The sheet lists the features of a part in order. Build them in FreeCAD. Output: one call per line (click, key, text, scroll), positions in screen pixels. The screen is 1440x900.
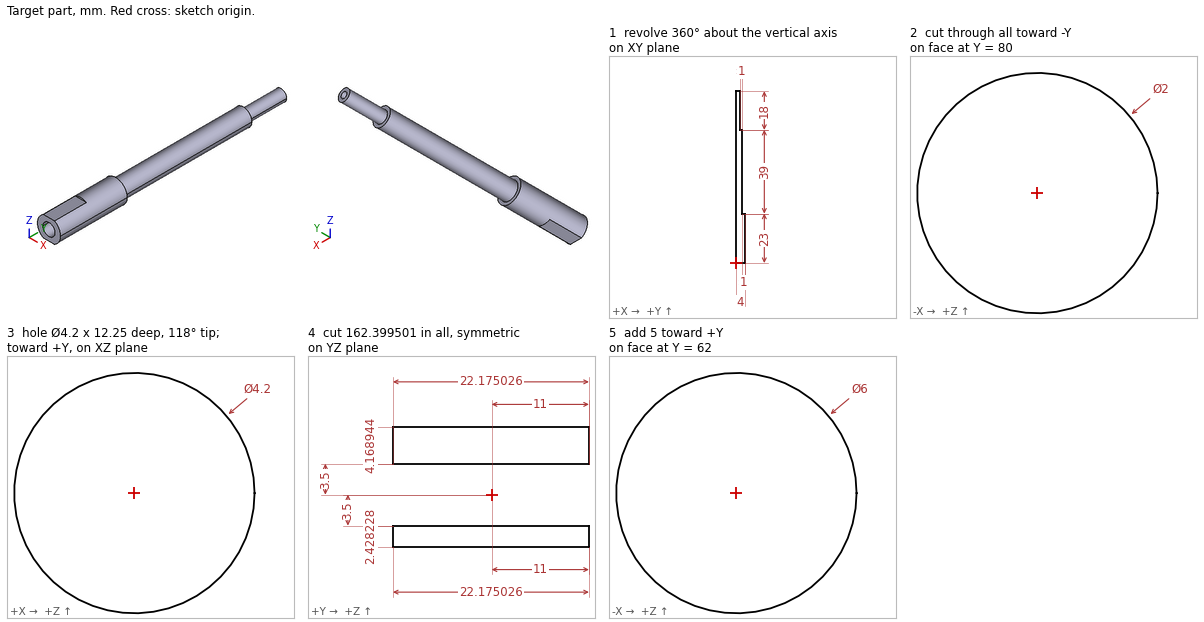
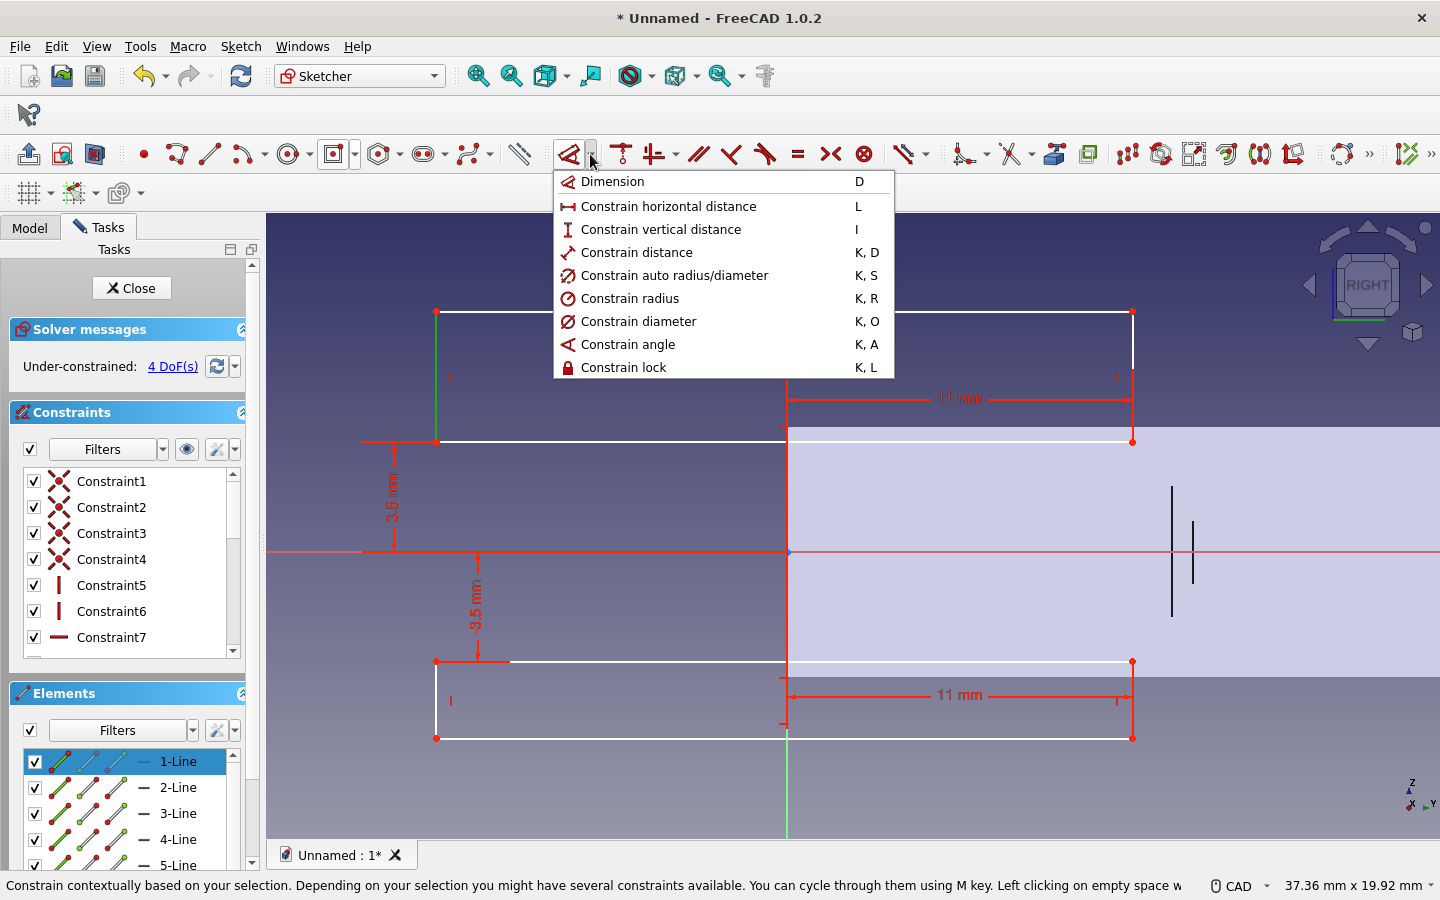
click(724, 230)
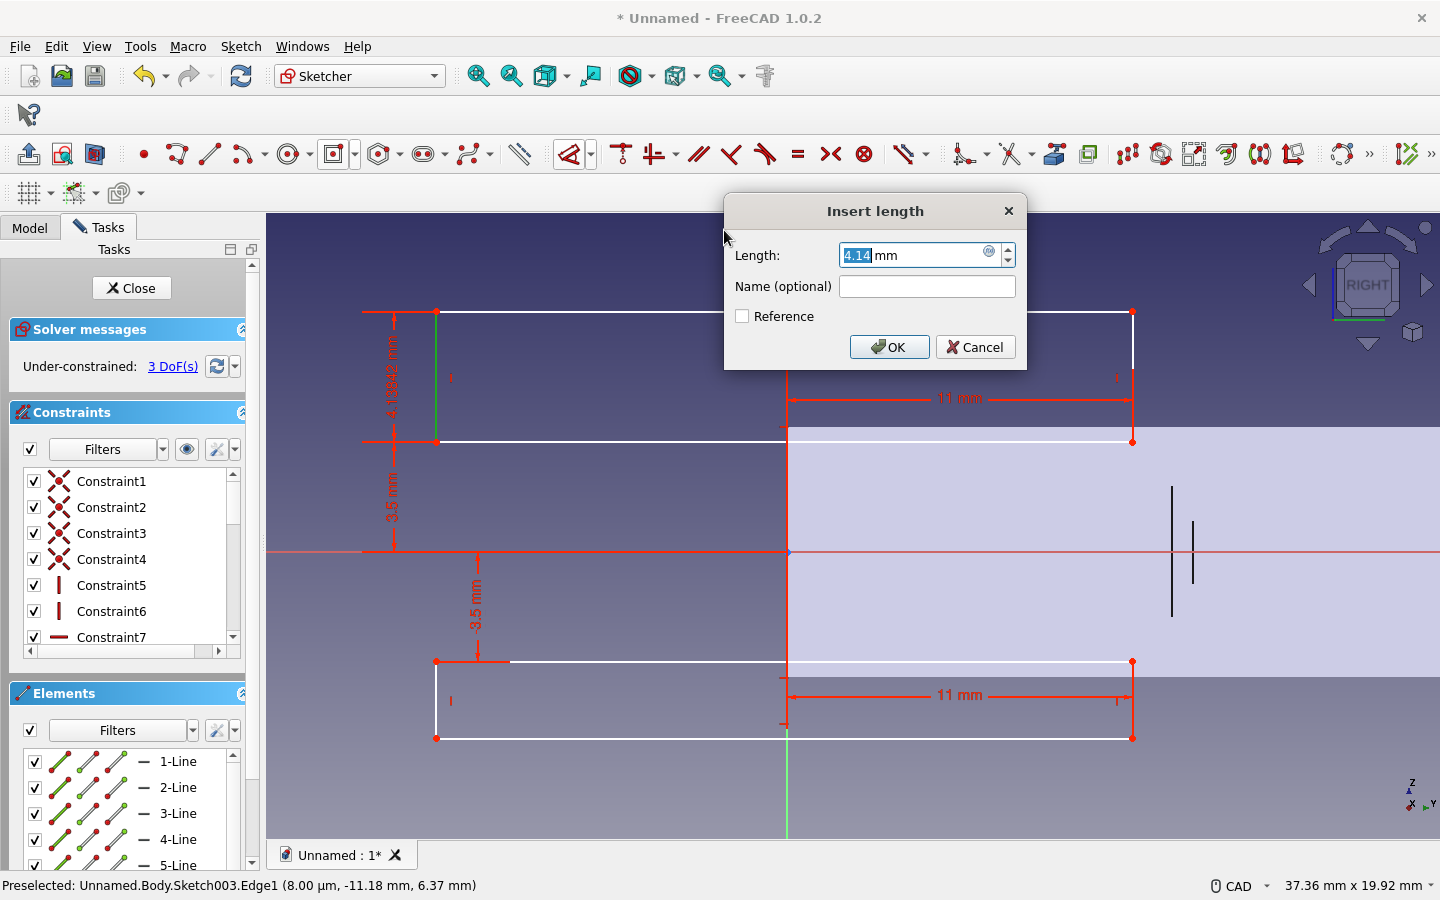
text(4.168944)
key(Return)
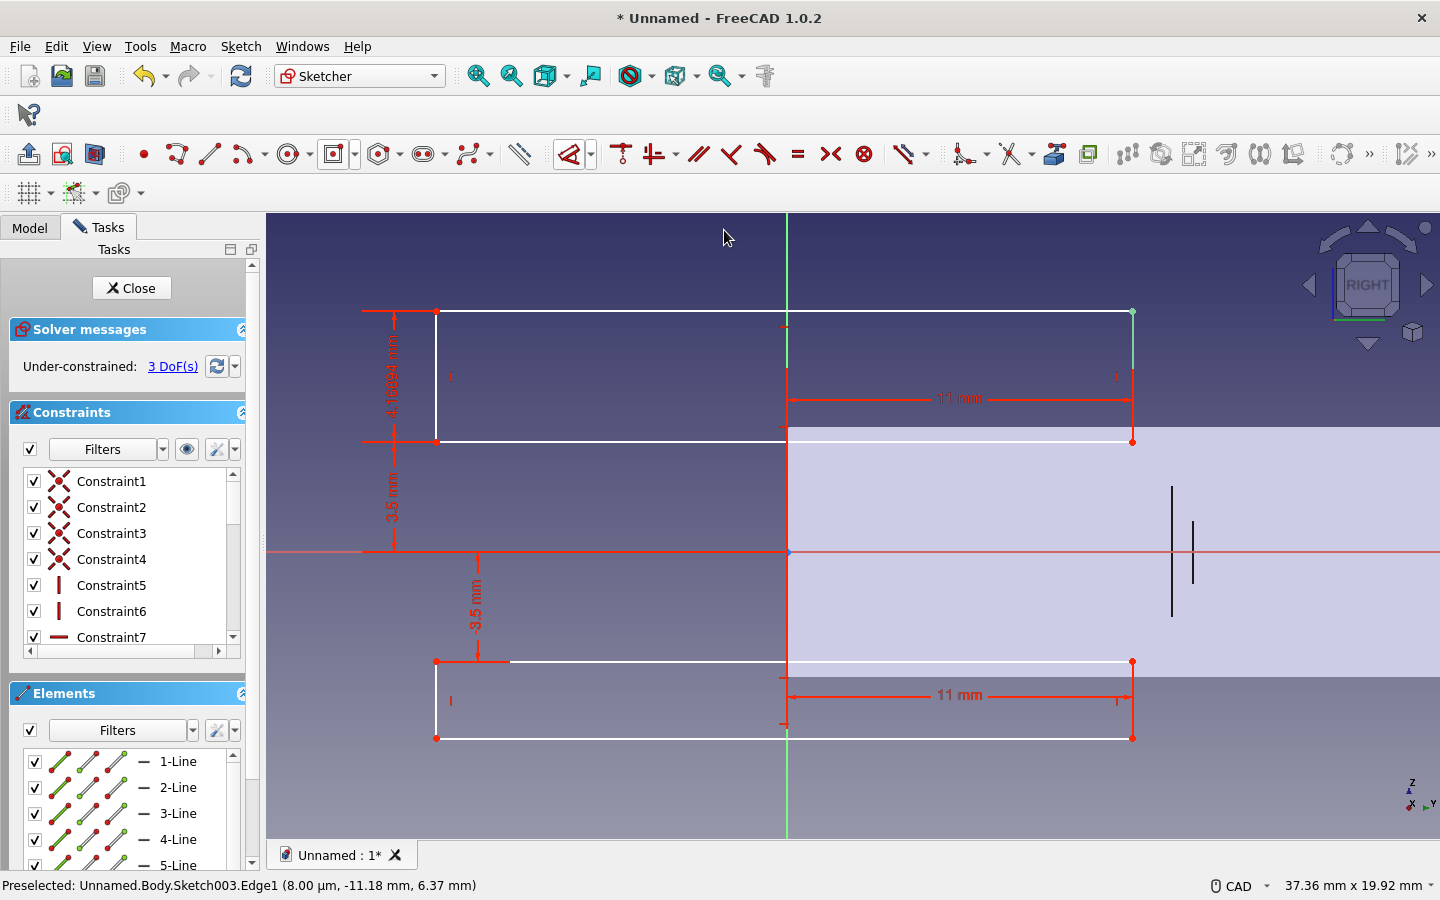
click(436, 685)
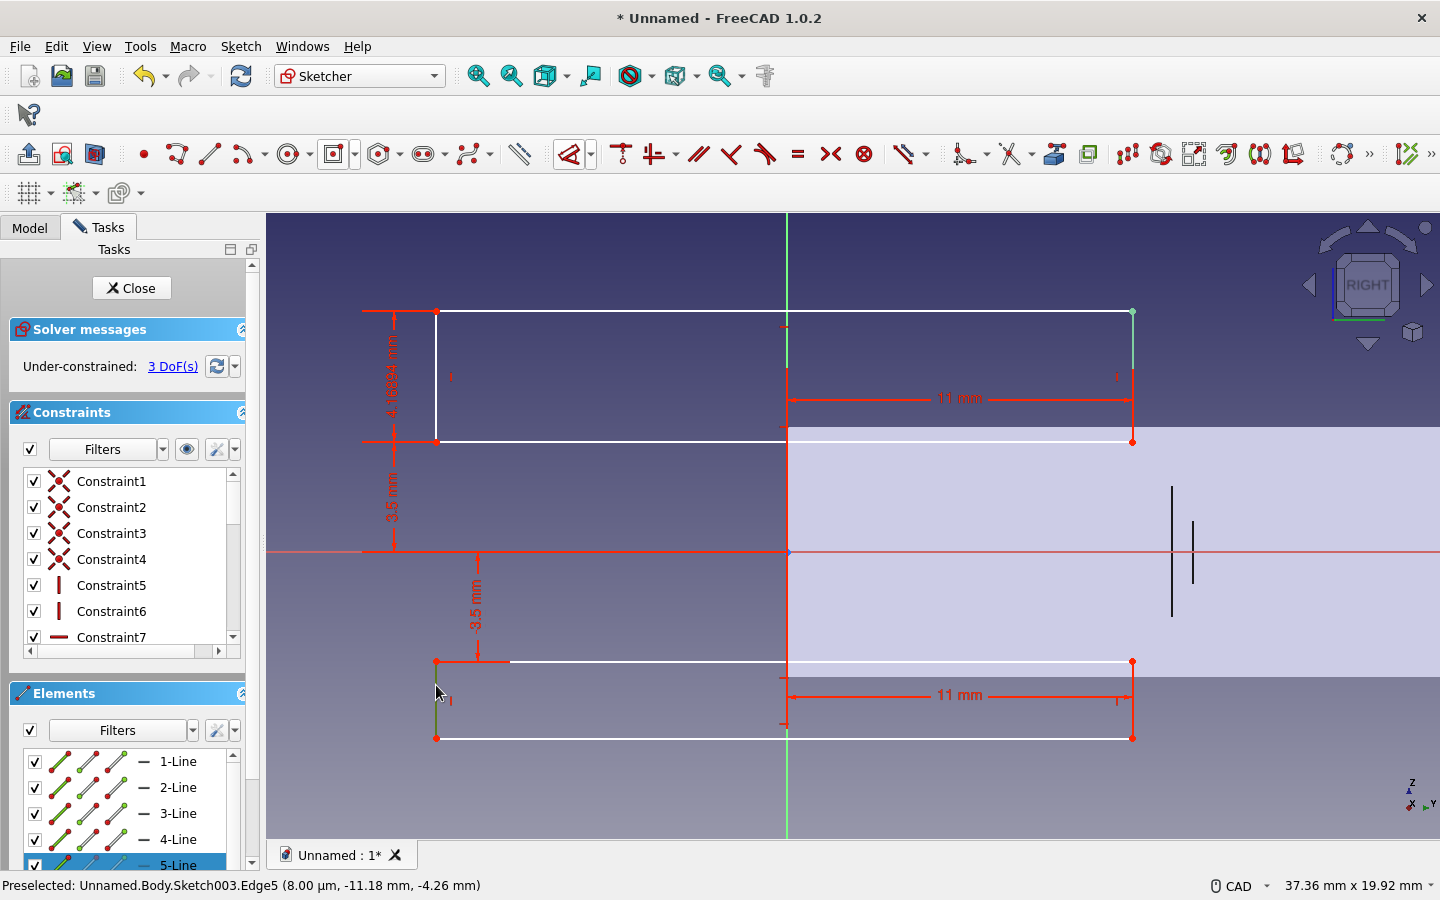
key(i)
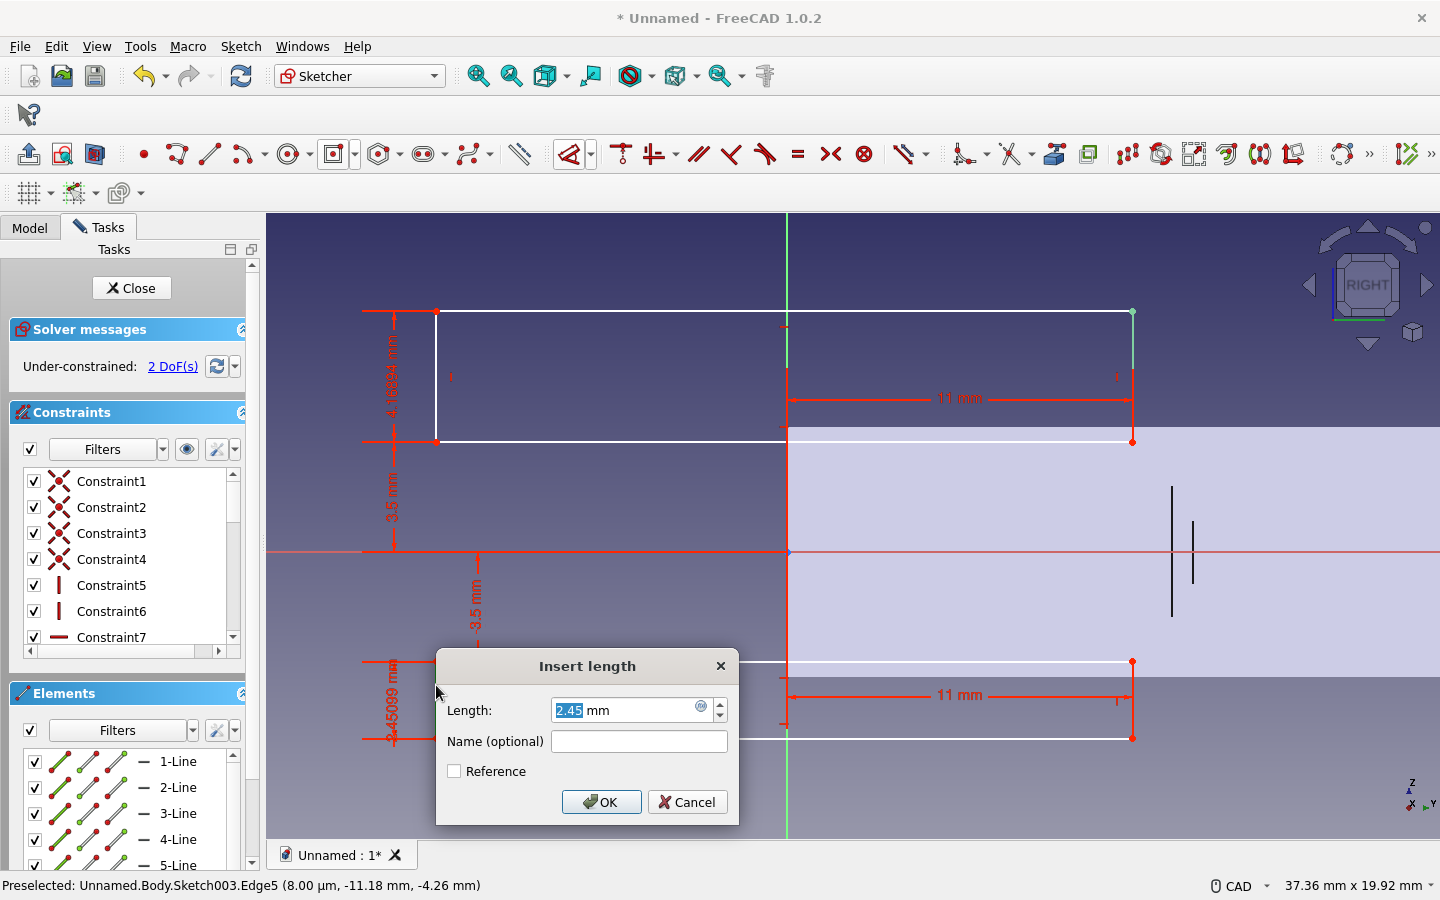
text(2.428228)
key(Return)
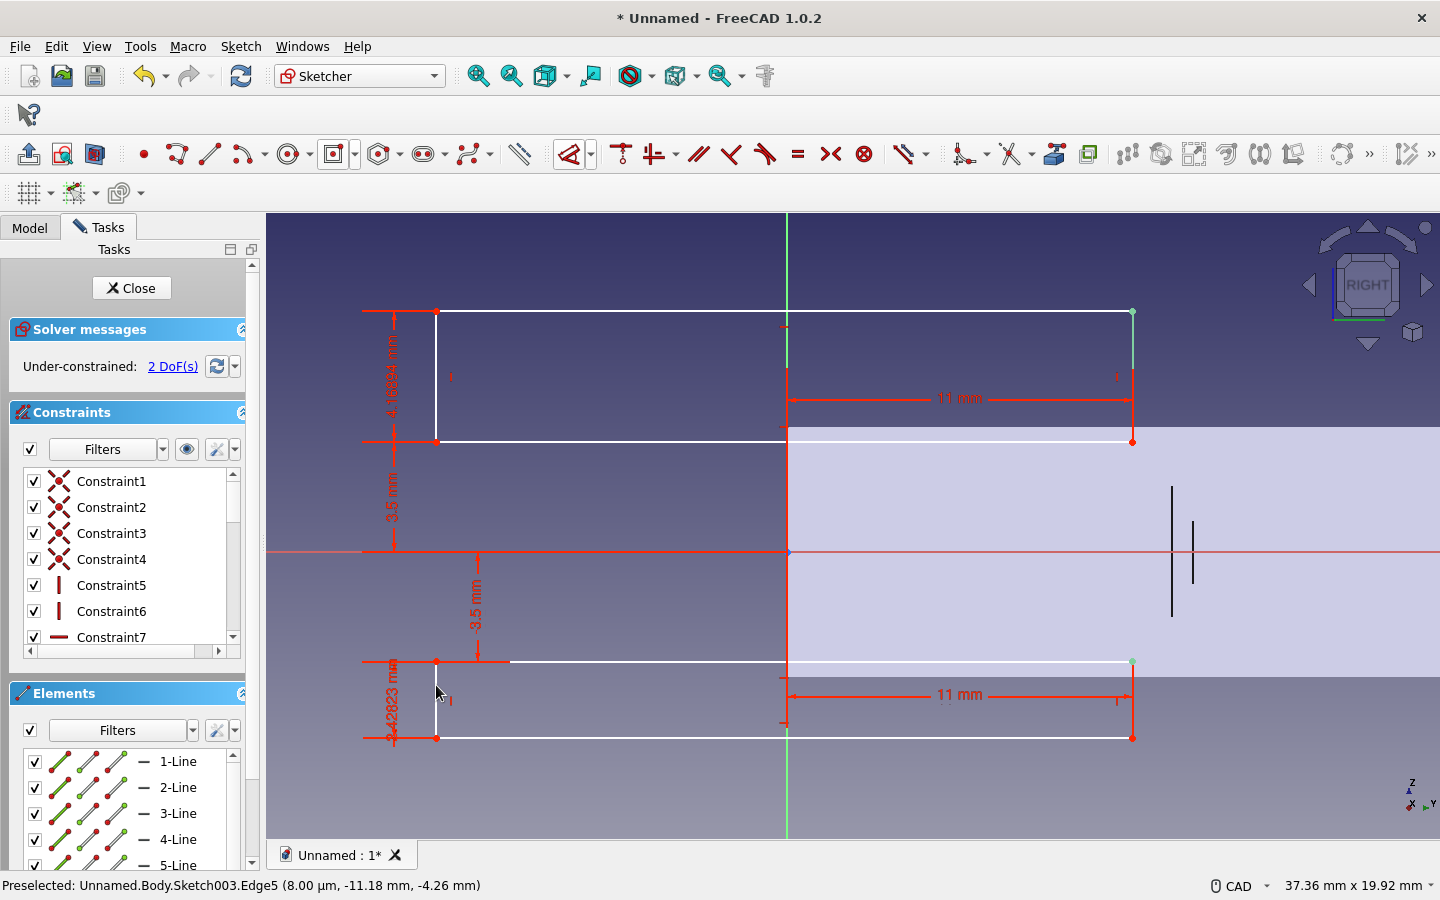
click(645, 442)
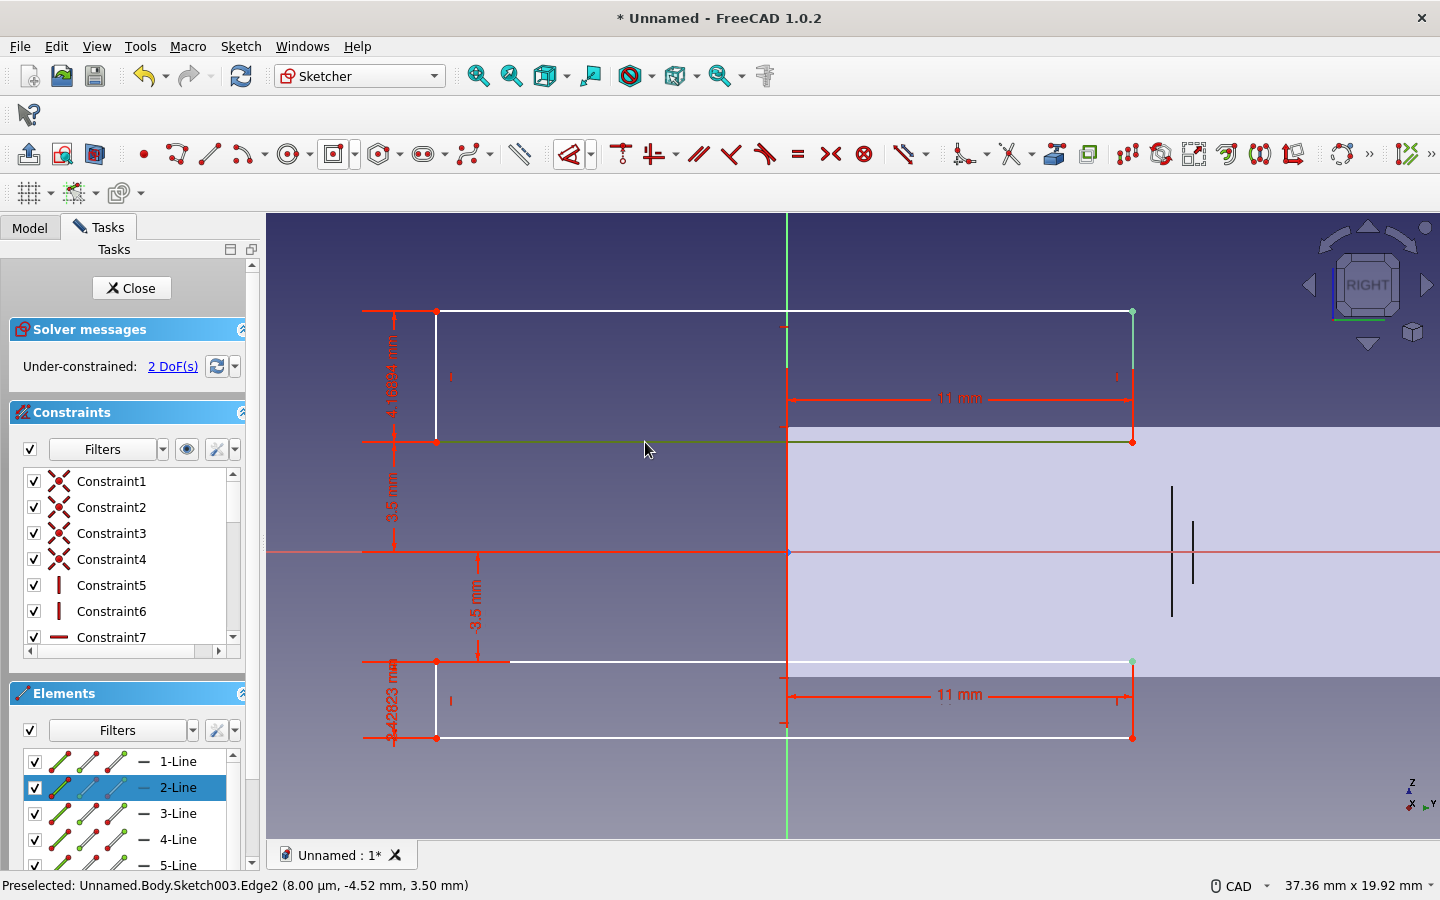
key(l)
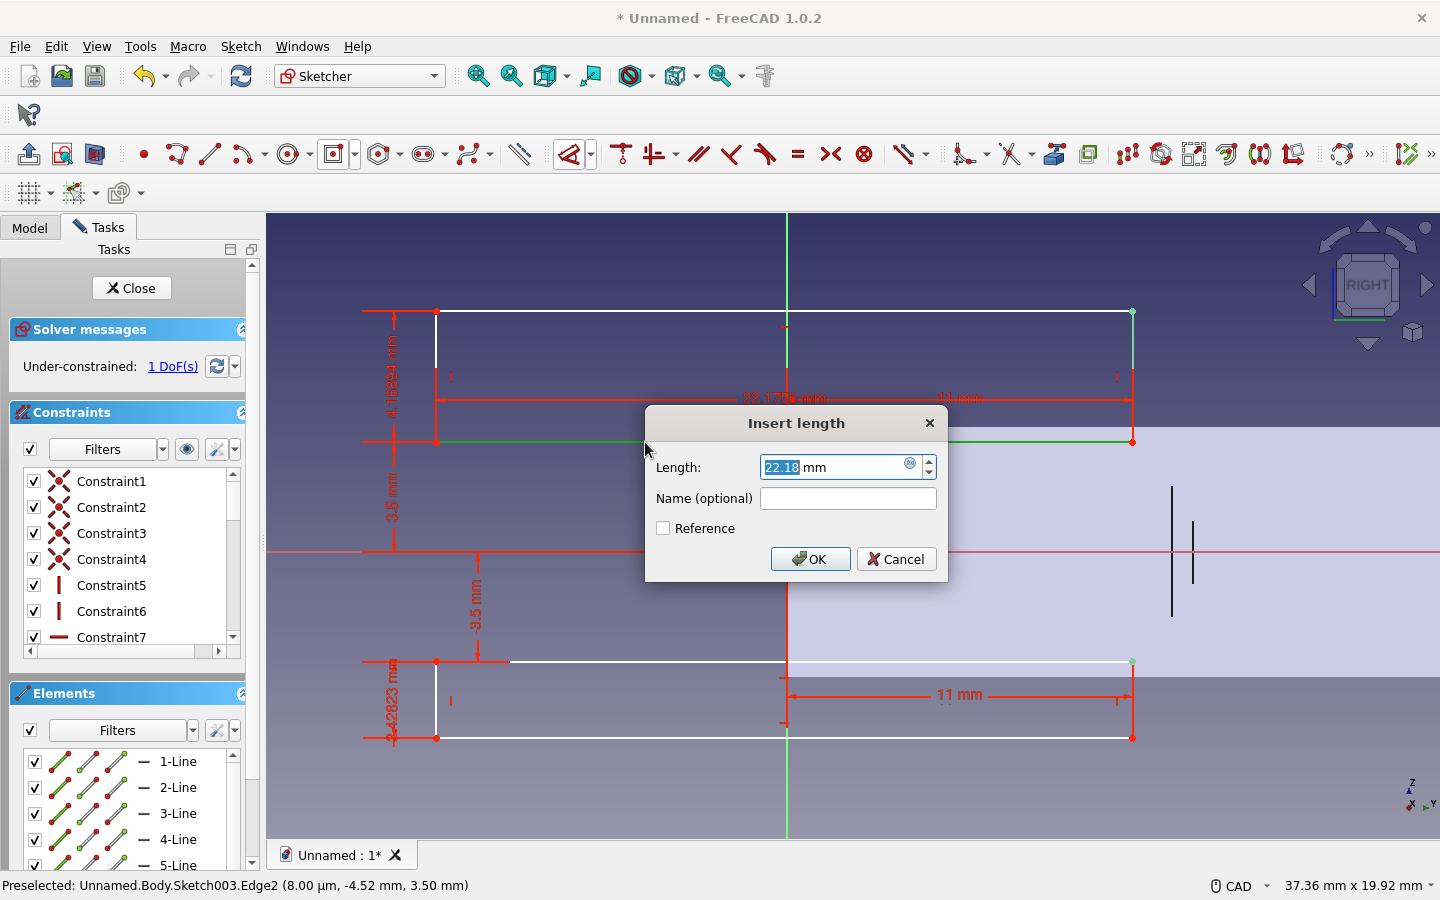
text(22.175026)
key(Return)